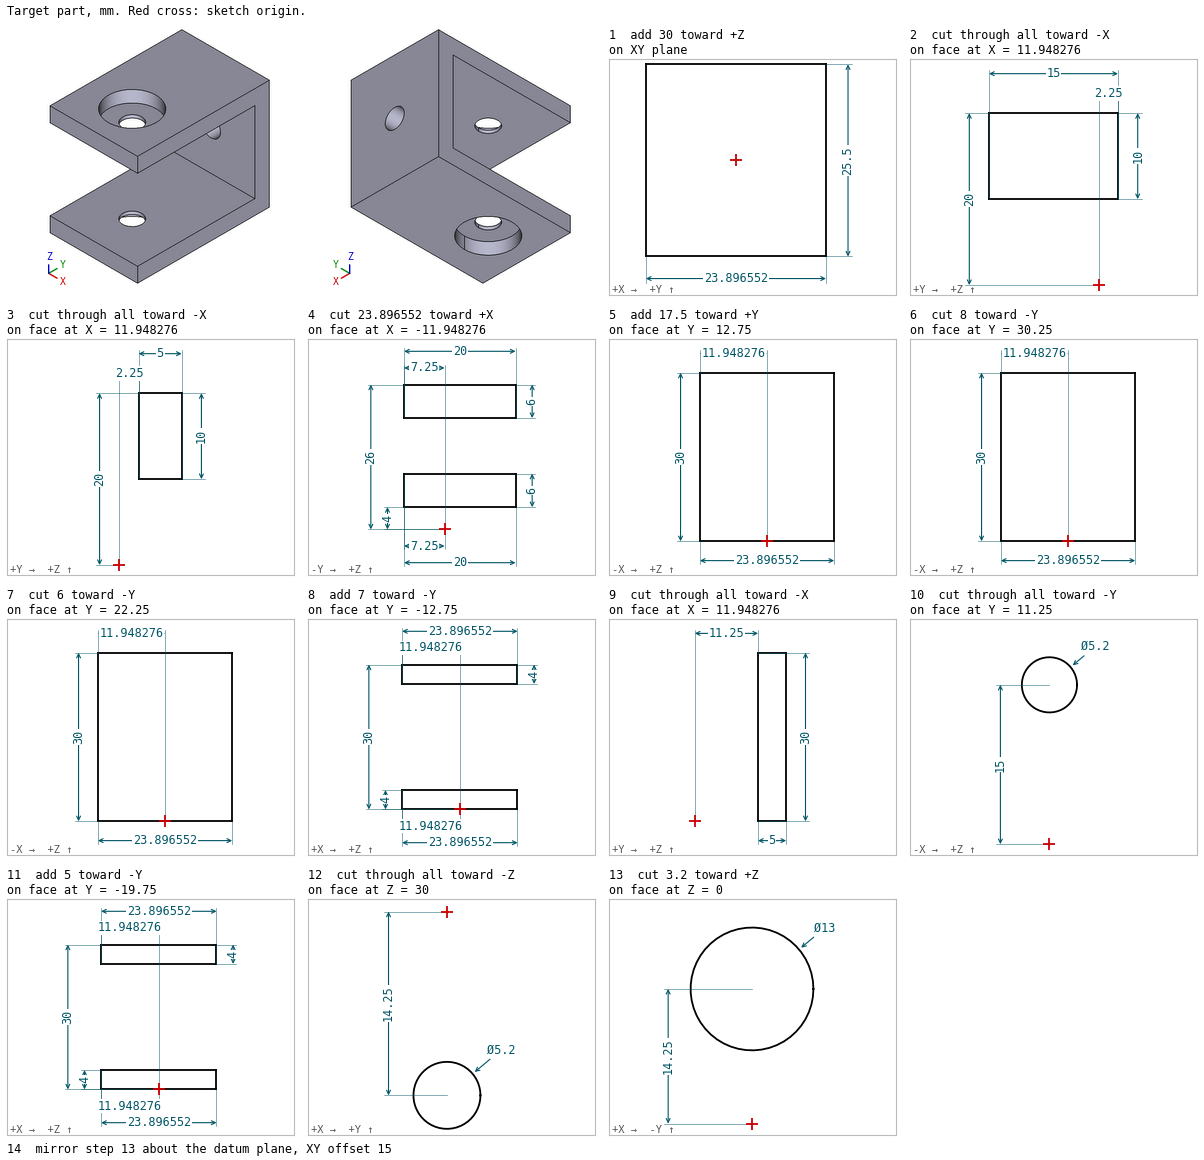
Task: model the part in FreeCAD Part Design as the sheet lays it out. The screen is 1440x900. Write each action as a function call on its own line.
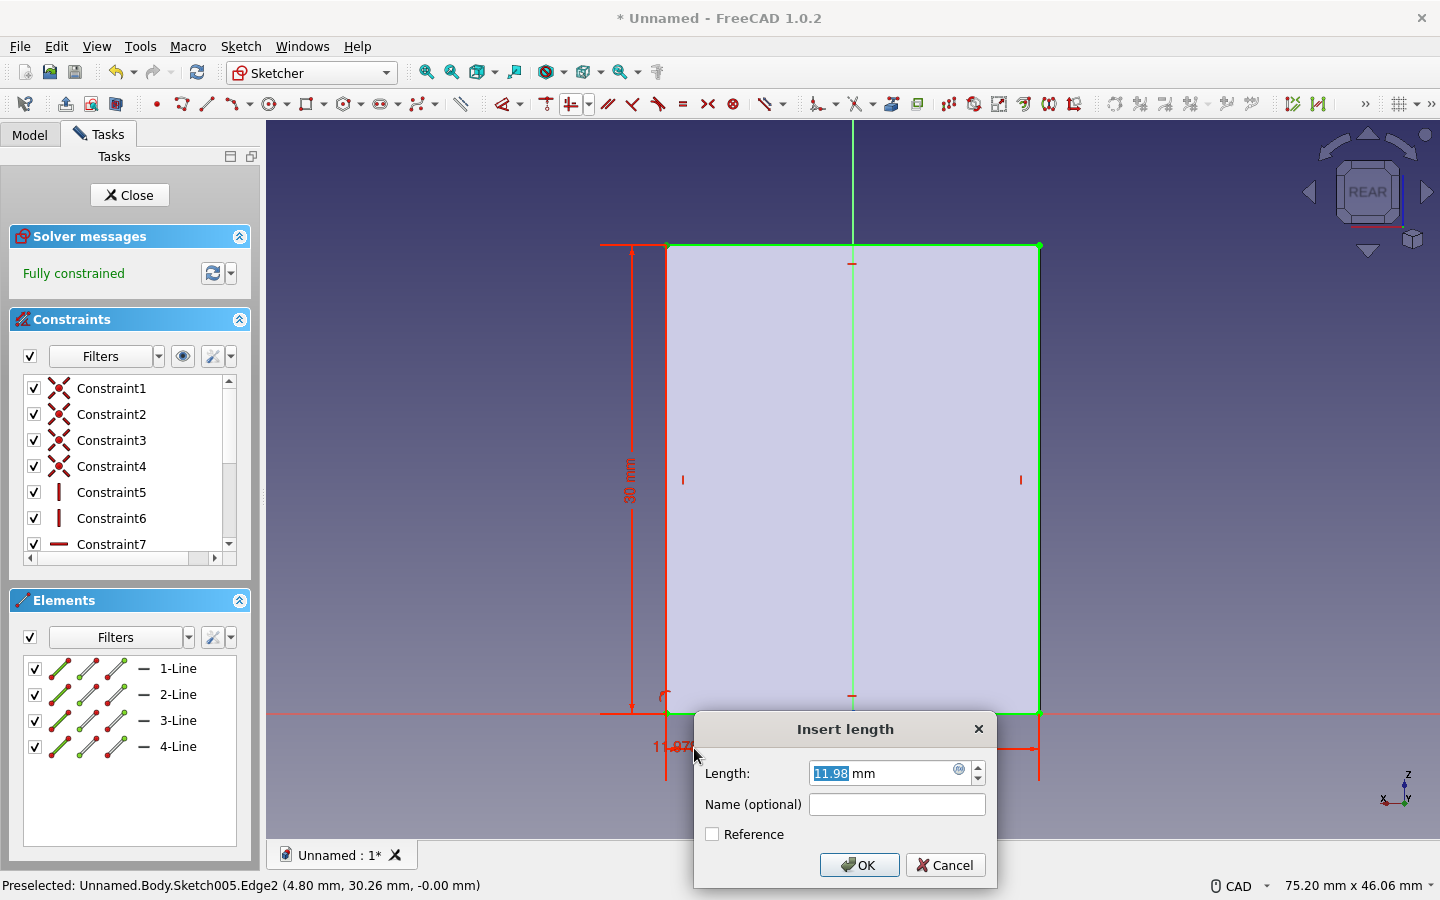
text(11.948276)
key(Return)
key(Escape)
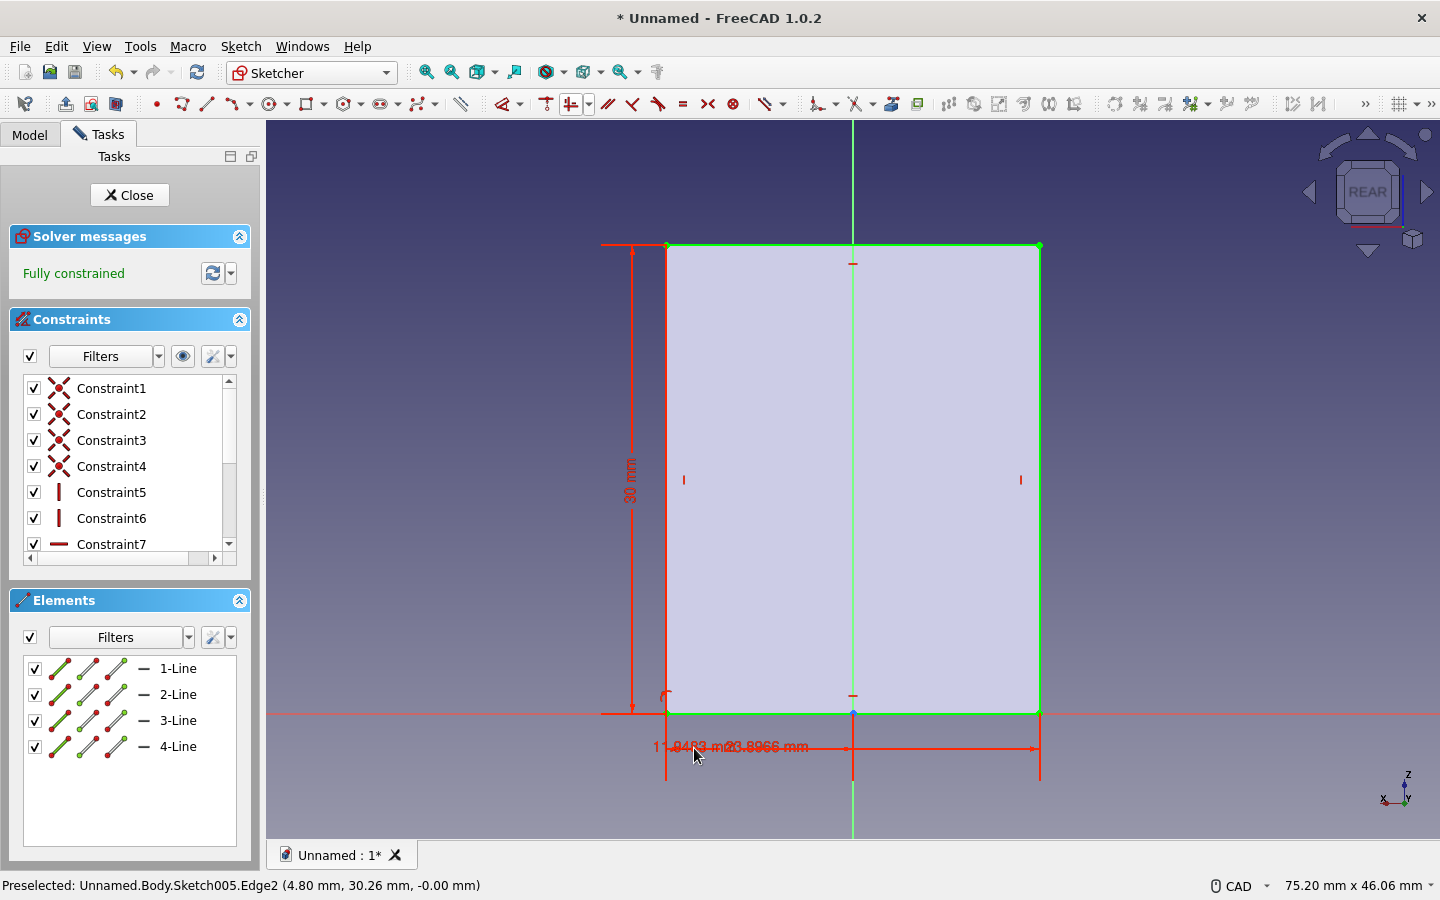
click(130, 195)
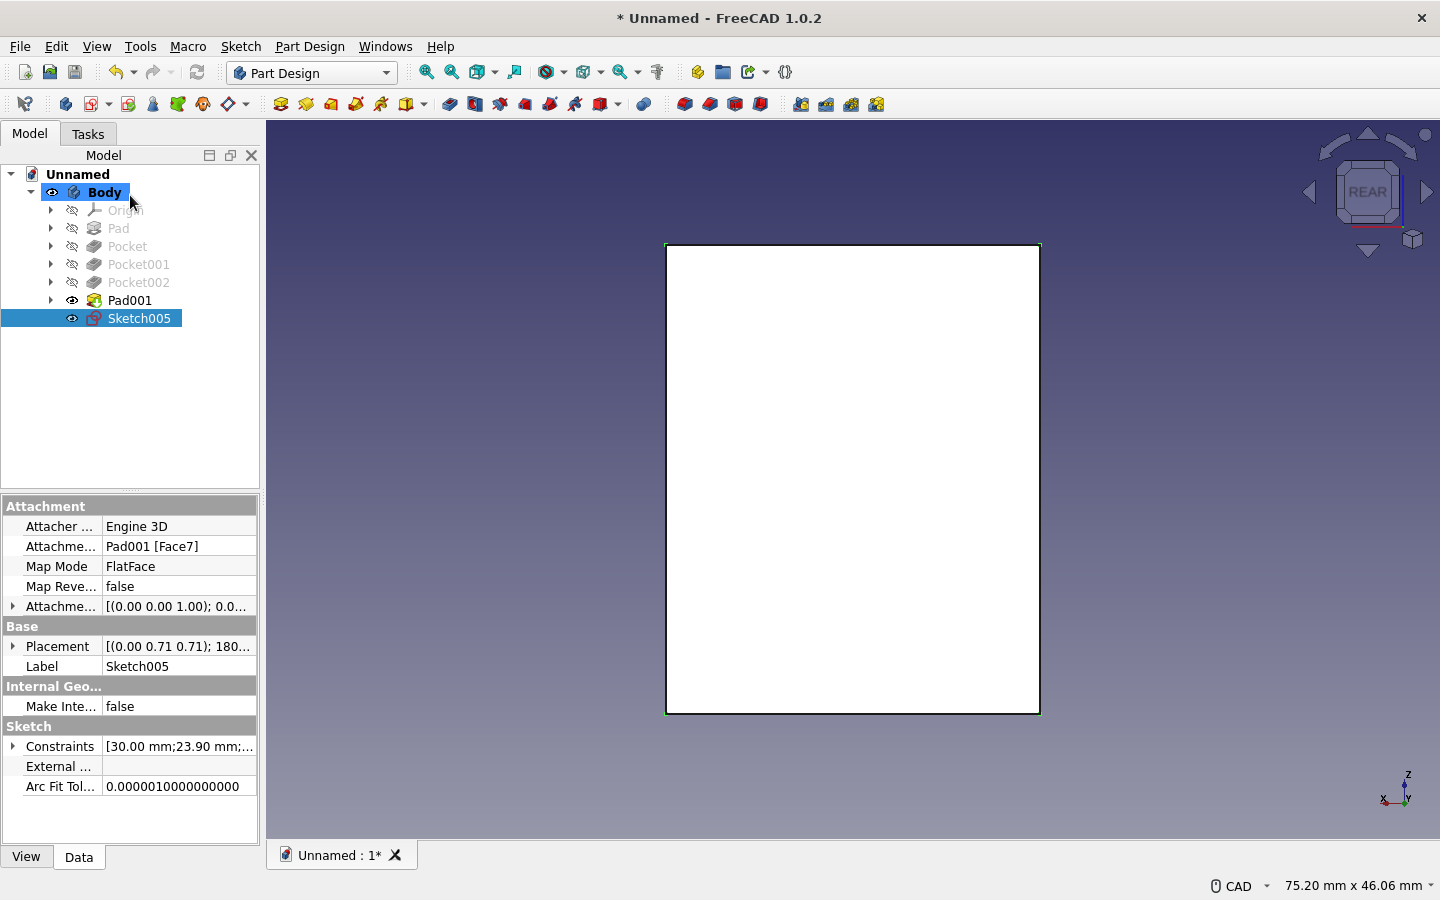
click(450, 104)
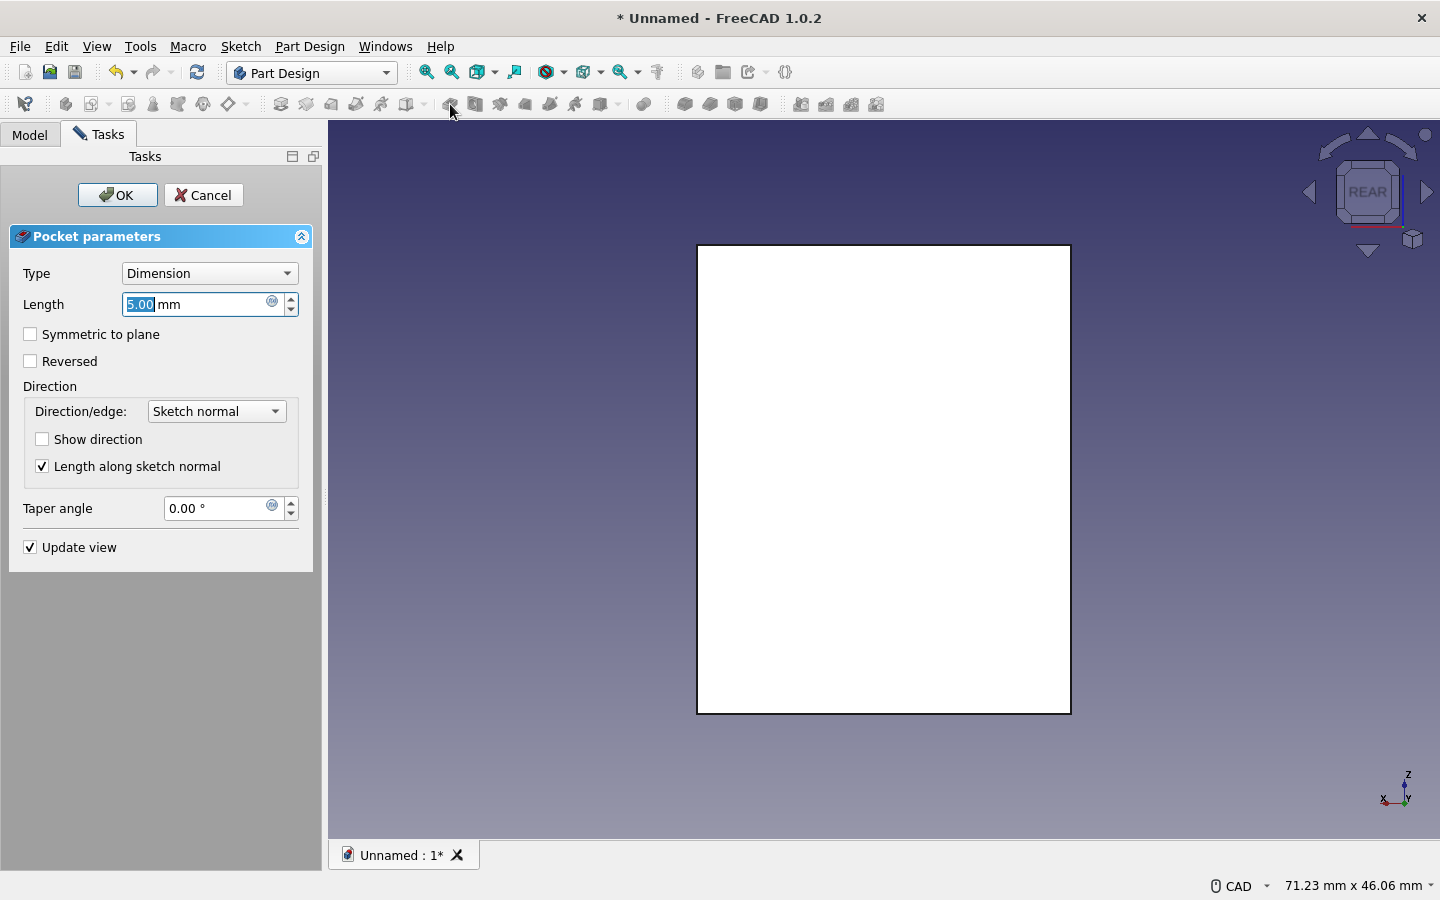
text(8)
key(Tab)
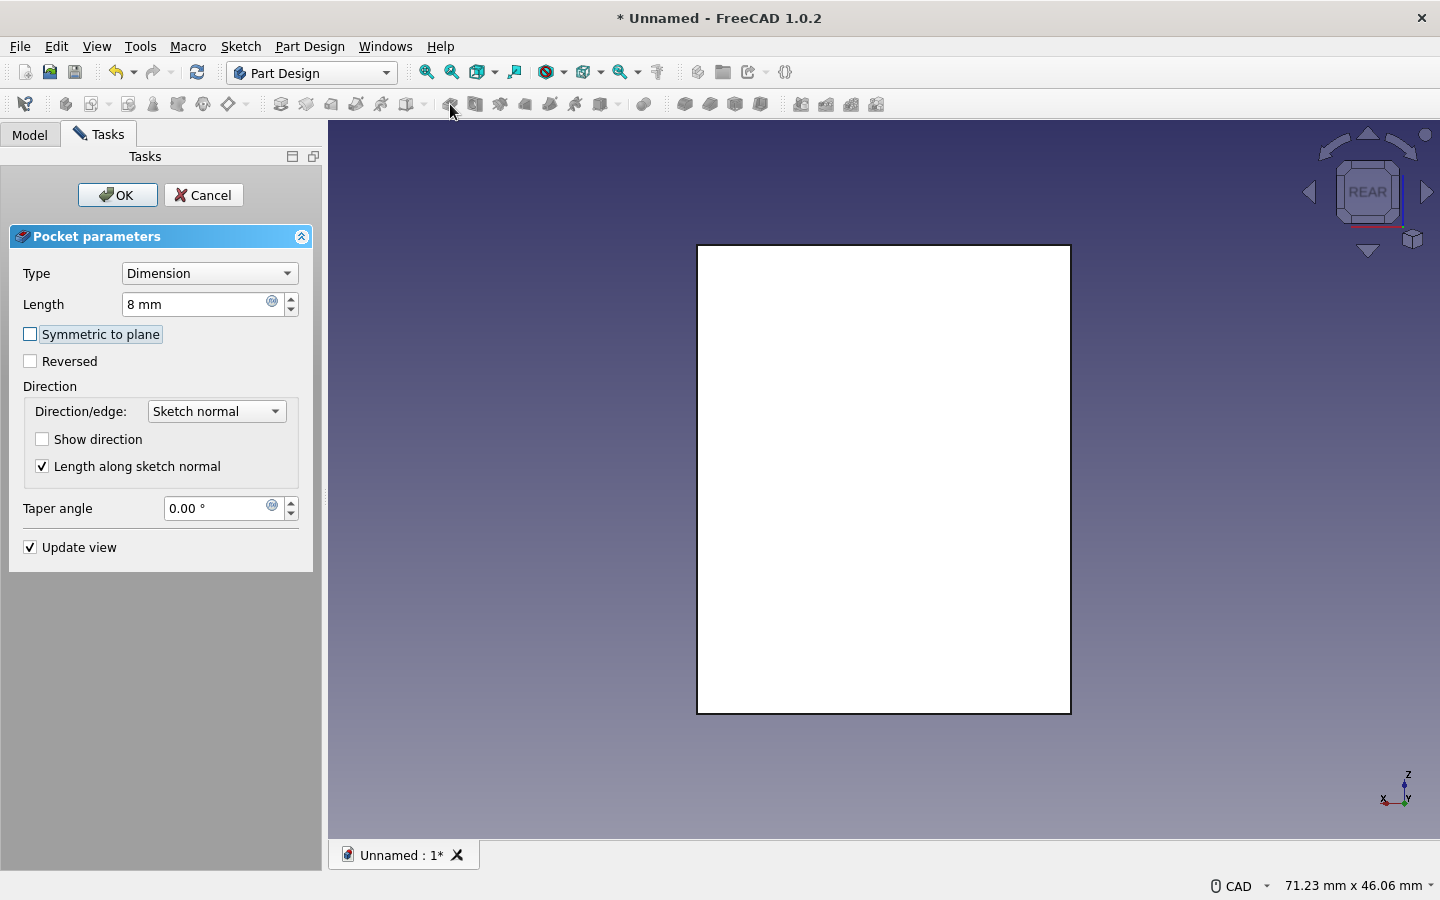
click(118, 195)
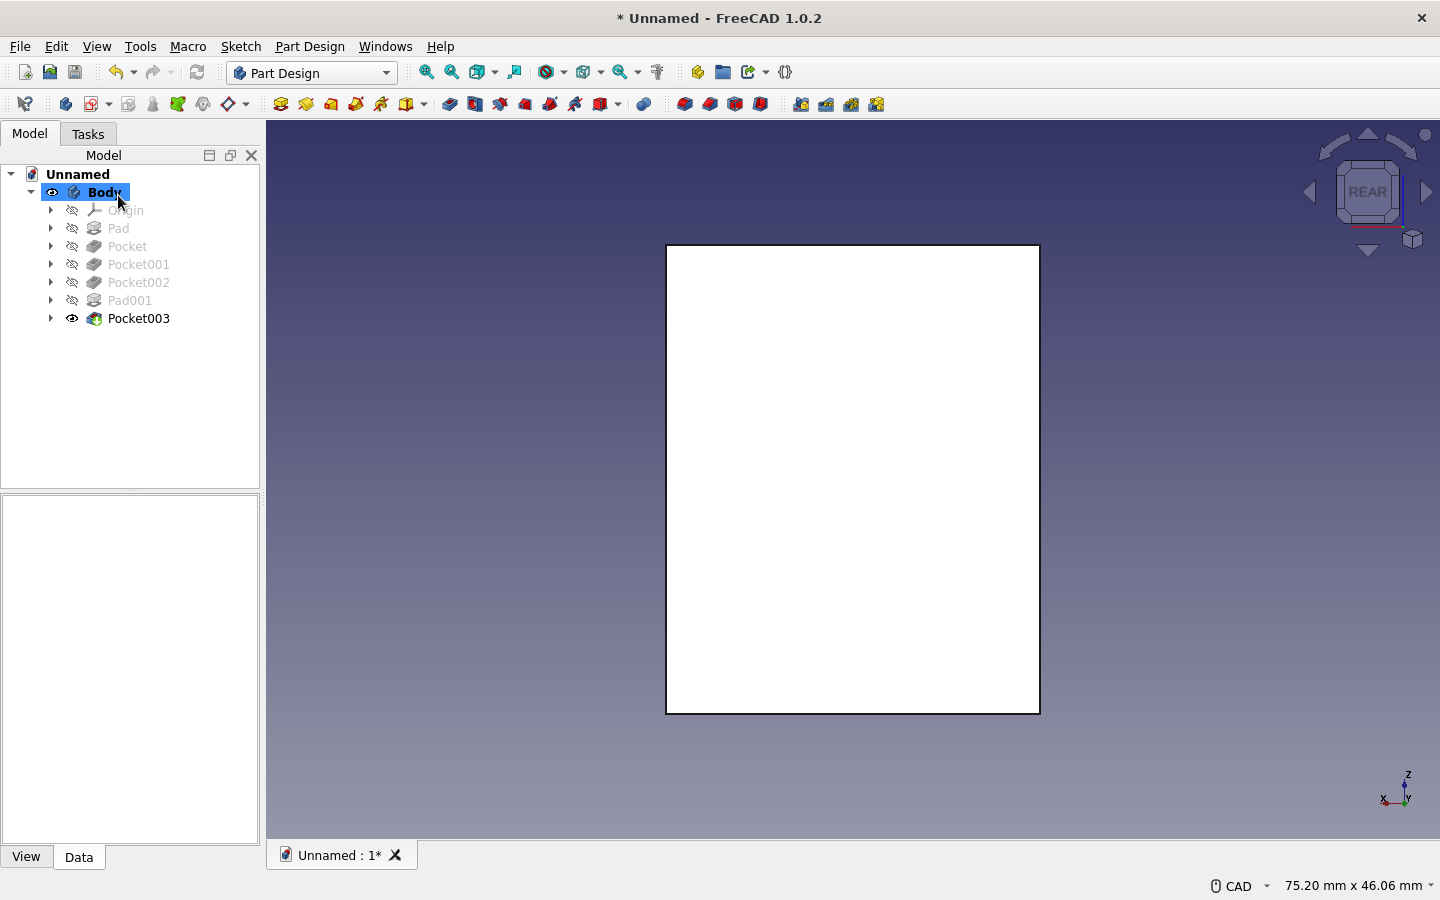
click(853, 479)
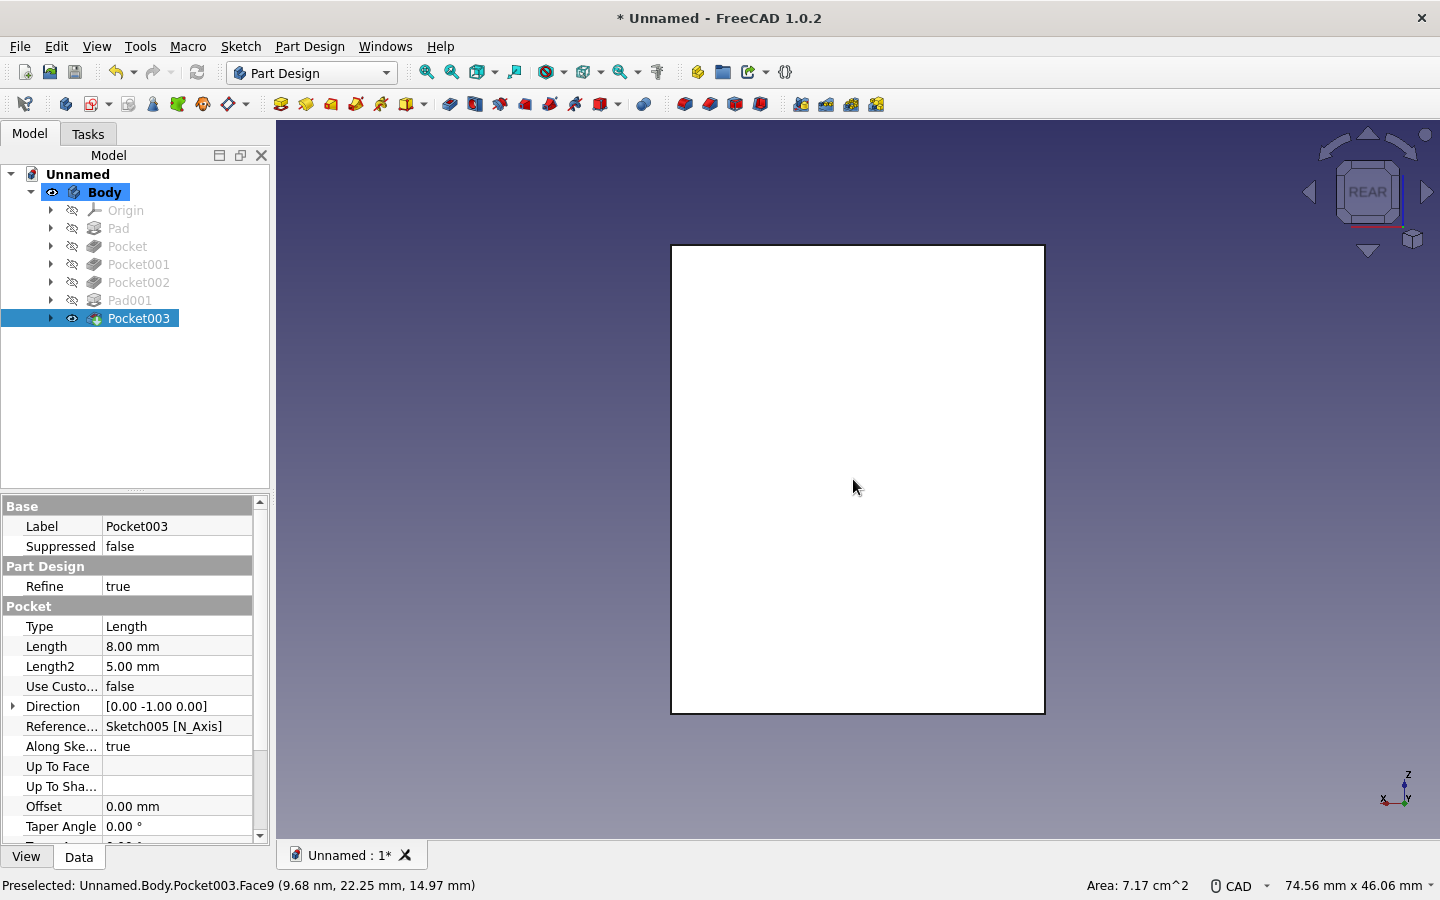
click(90, 104)